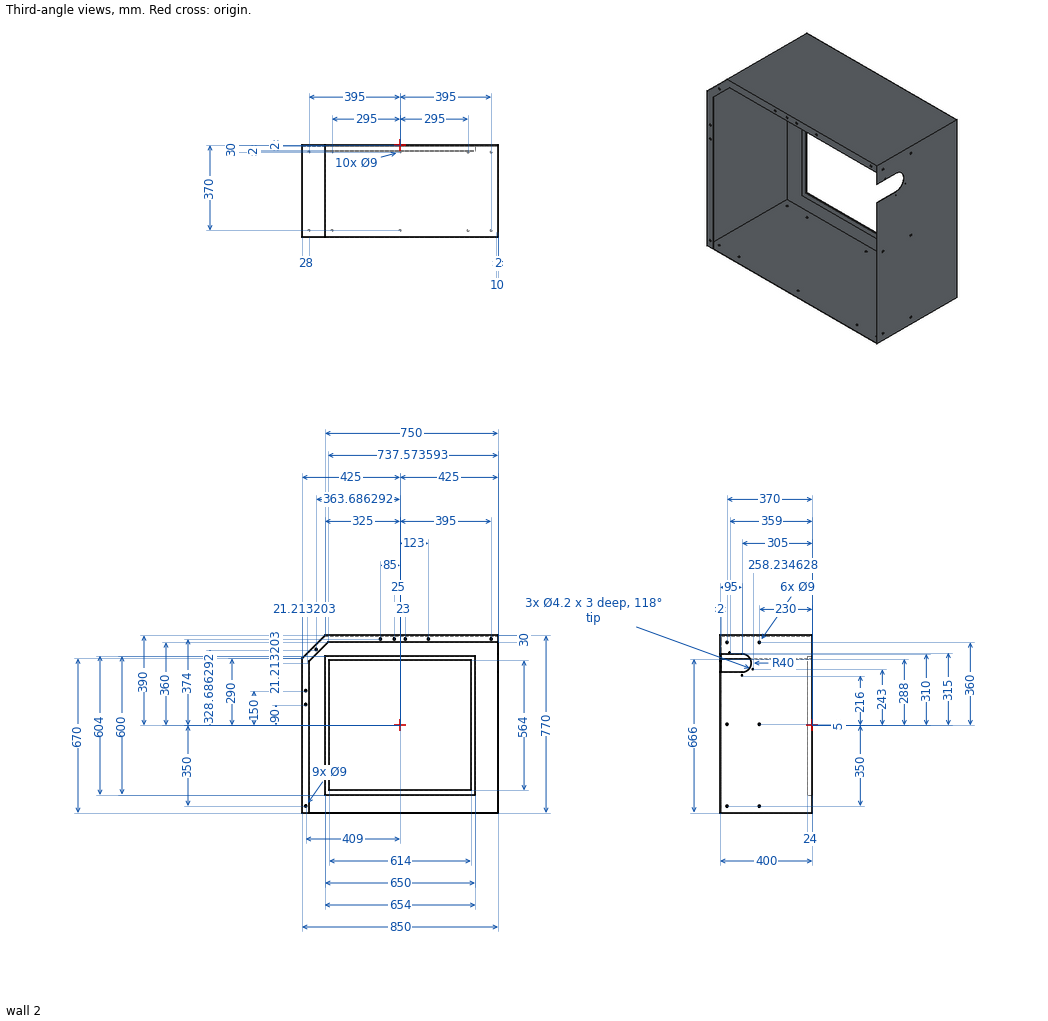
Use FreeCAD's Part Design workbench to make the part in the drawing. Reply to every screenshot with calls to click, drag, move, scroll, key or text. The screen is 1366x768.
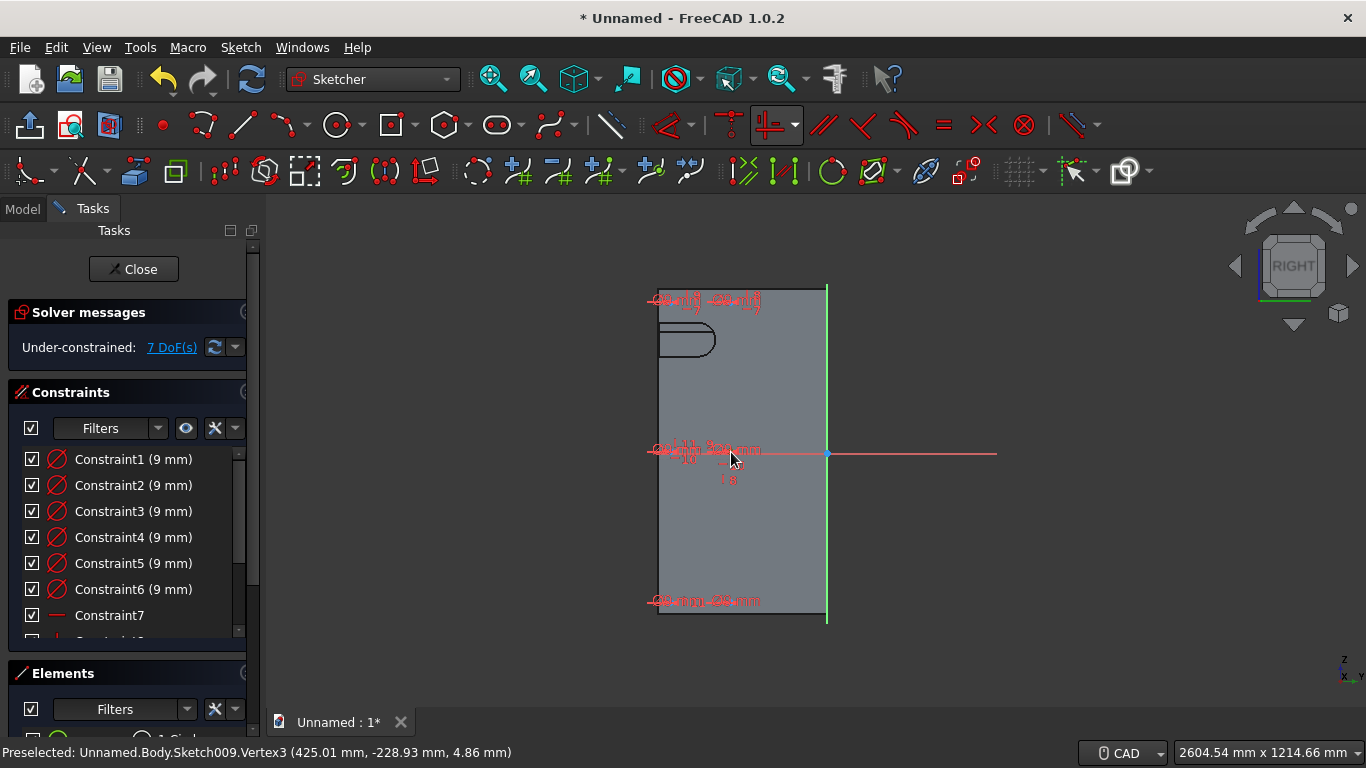
click(730, 603)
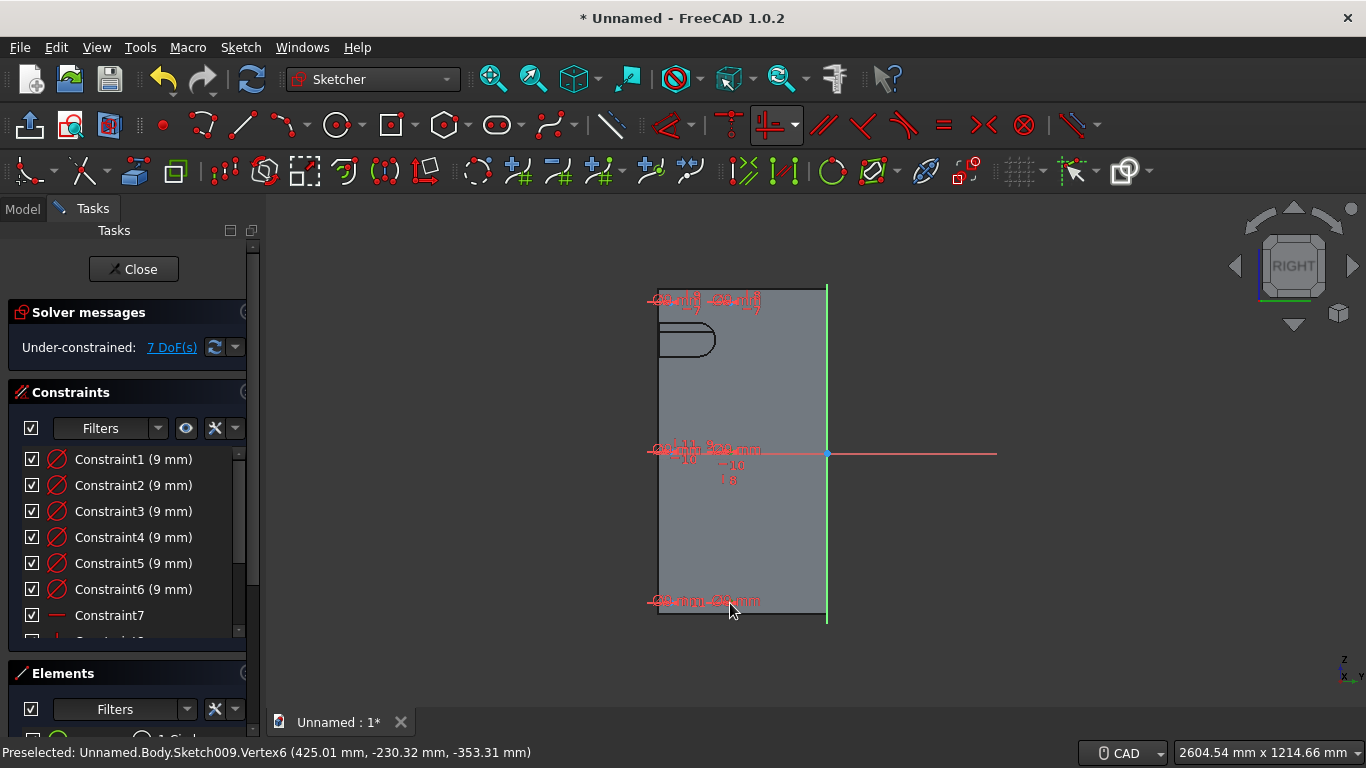
click(798, 126)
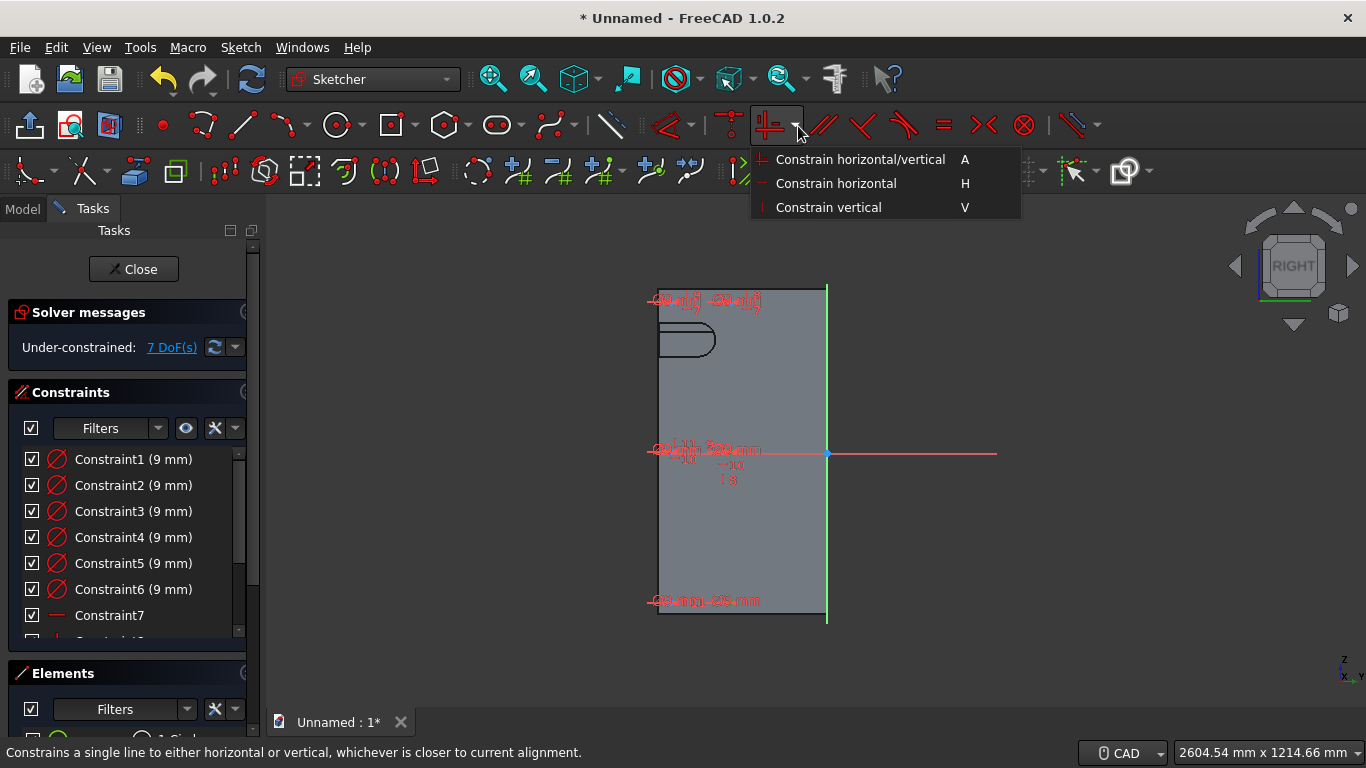
click(886, 207)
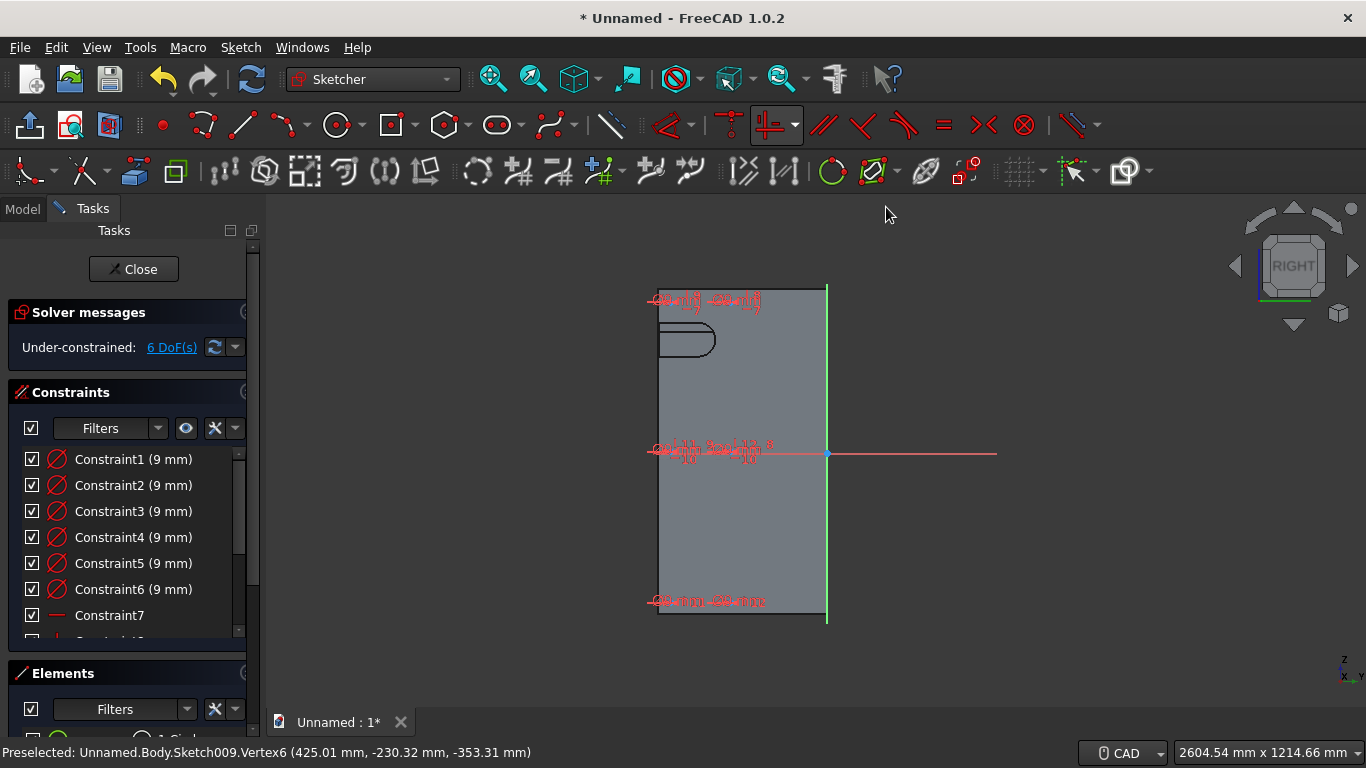
click(671, 603)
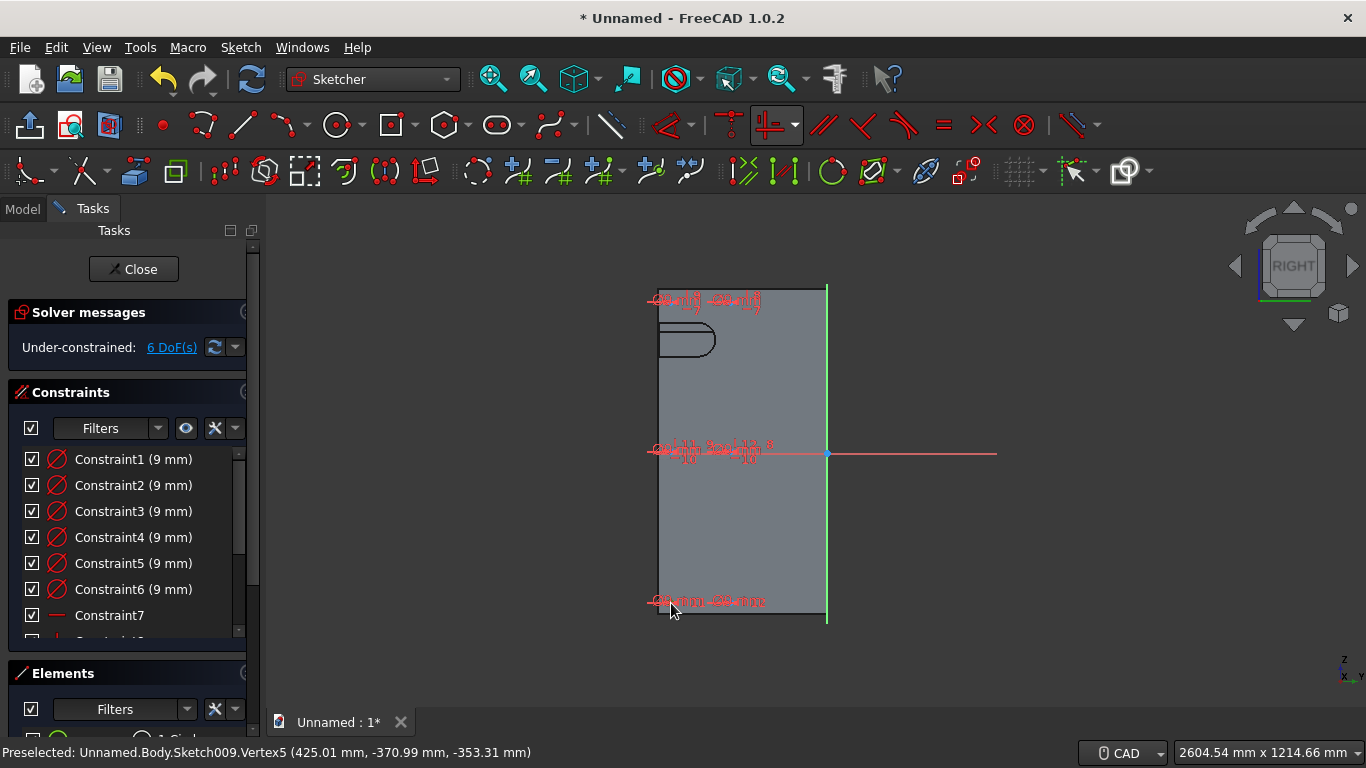
click(731, 603)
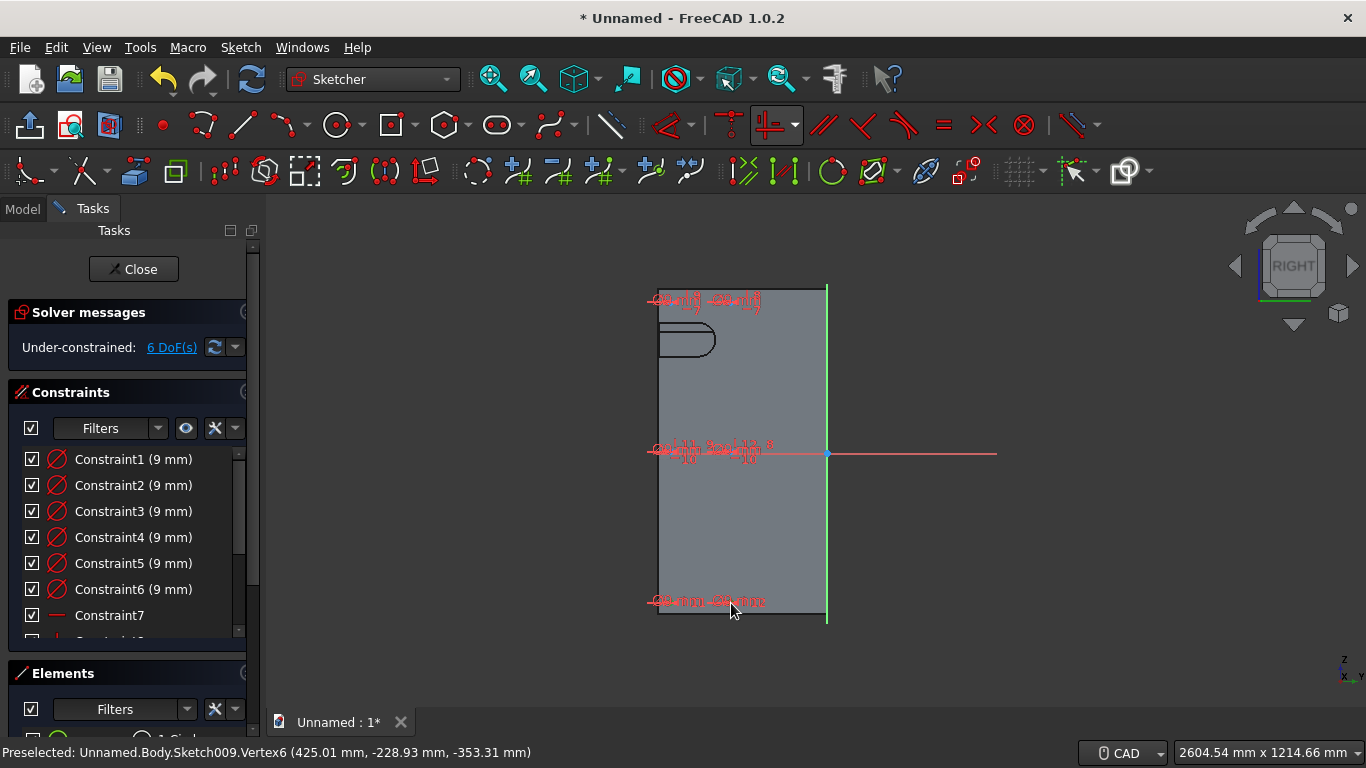
click(798, 126)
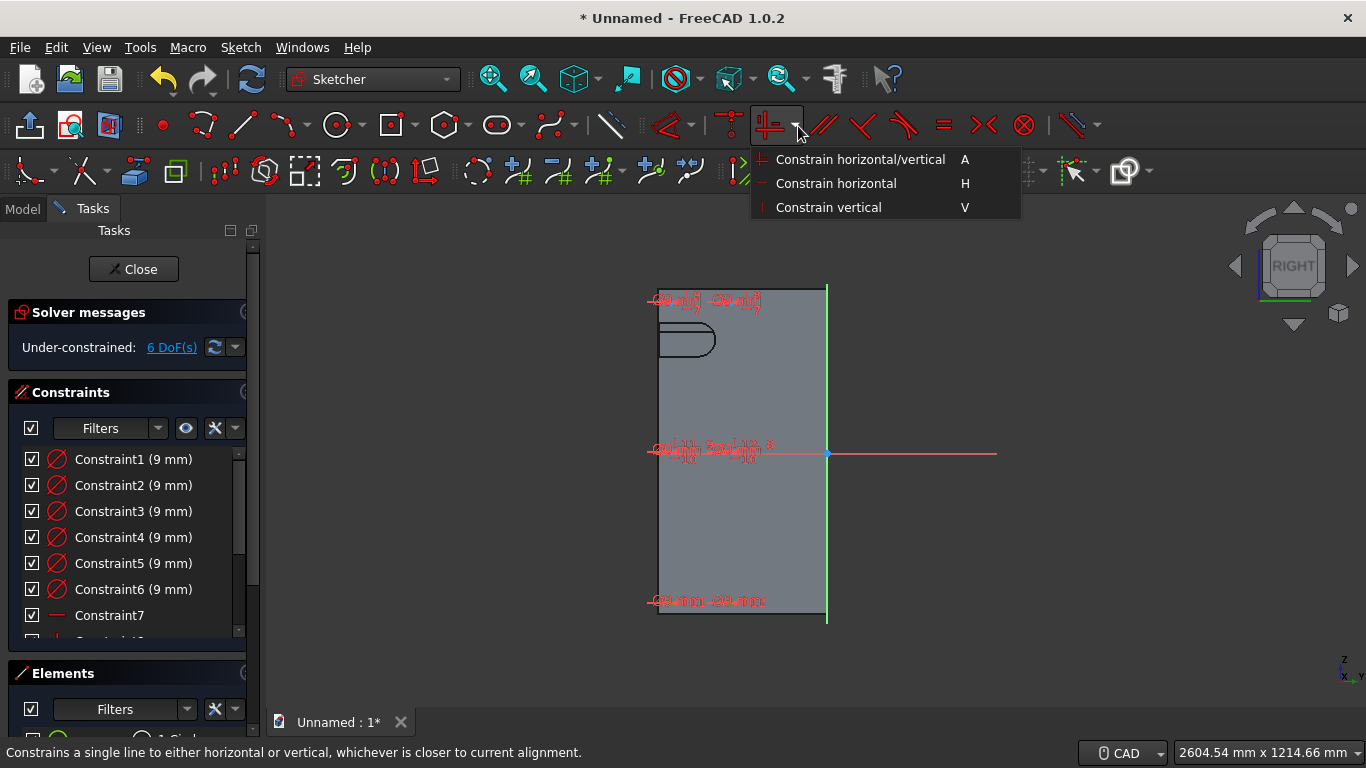
click(886, 183)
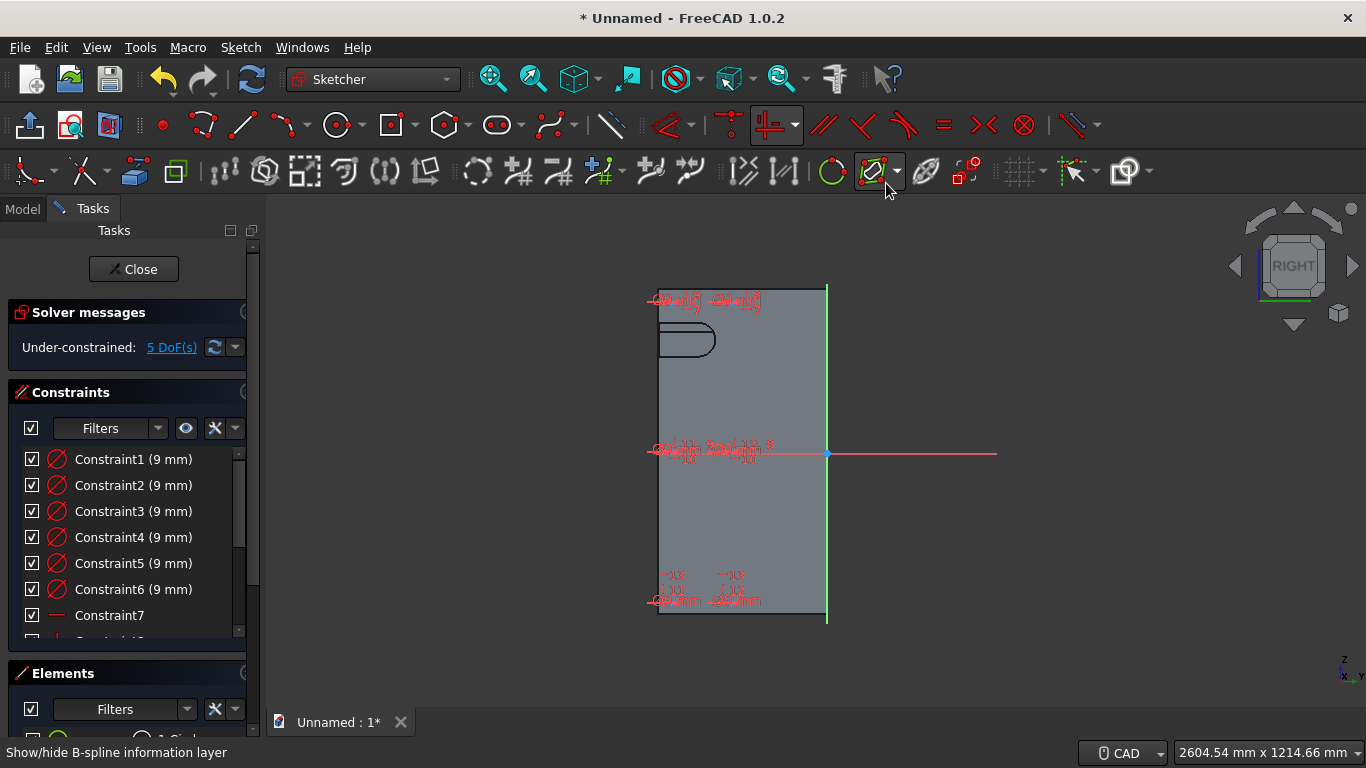
click(666, 126)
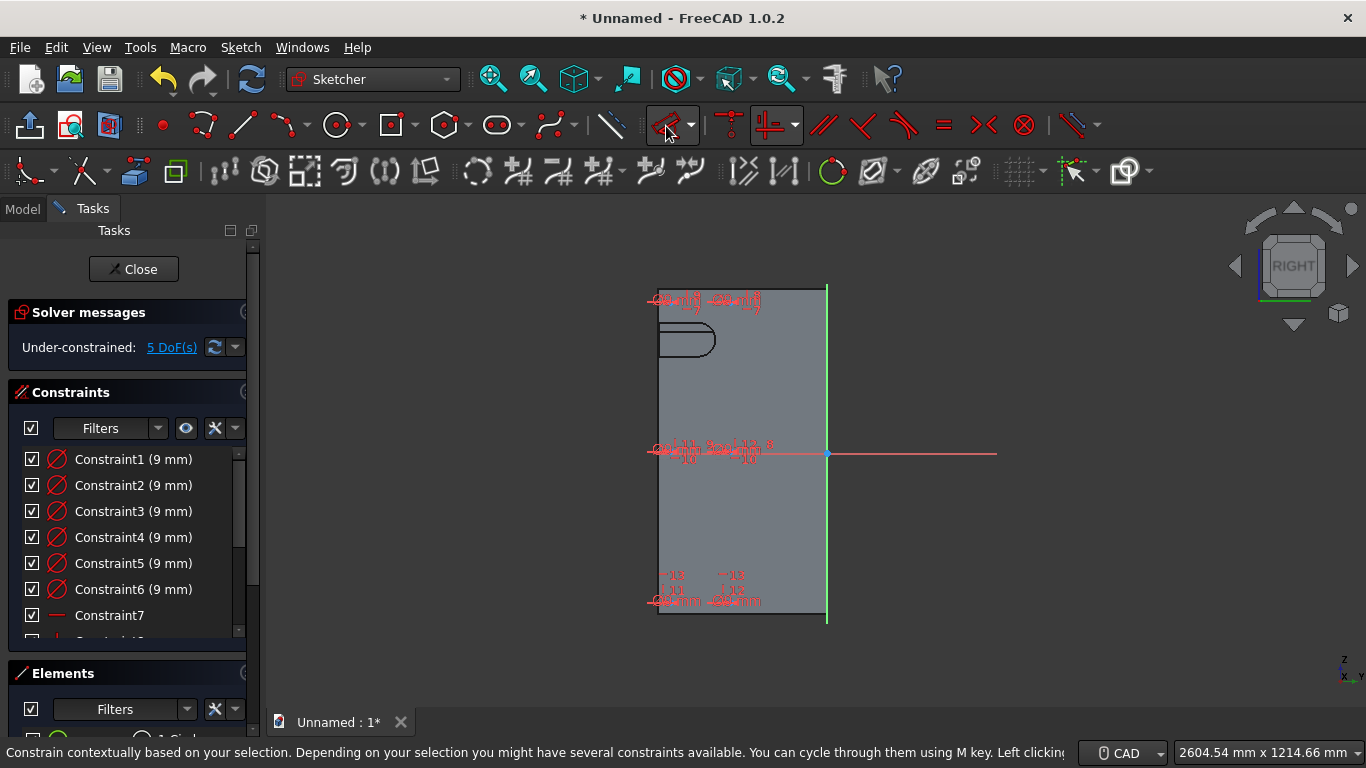
scroll(731, 452, up, 15)